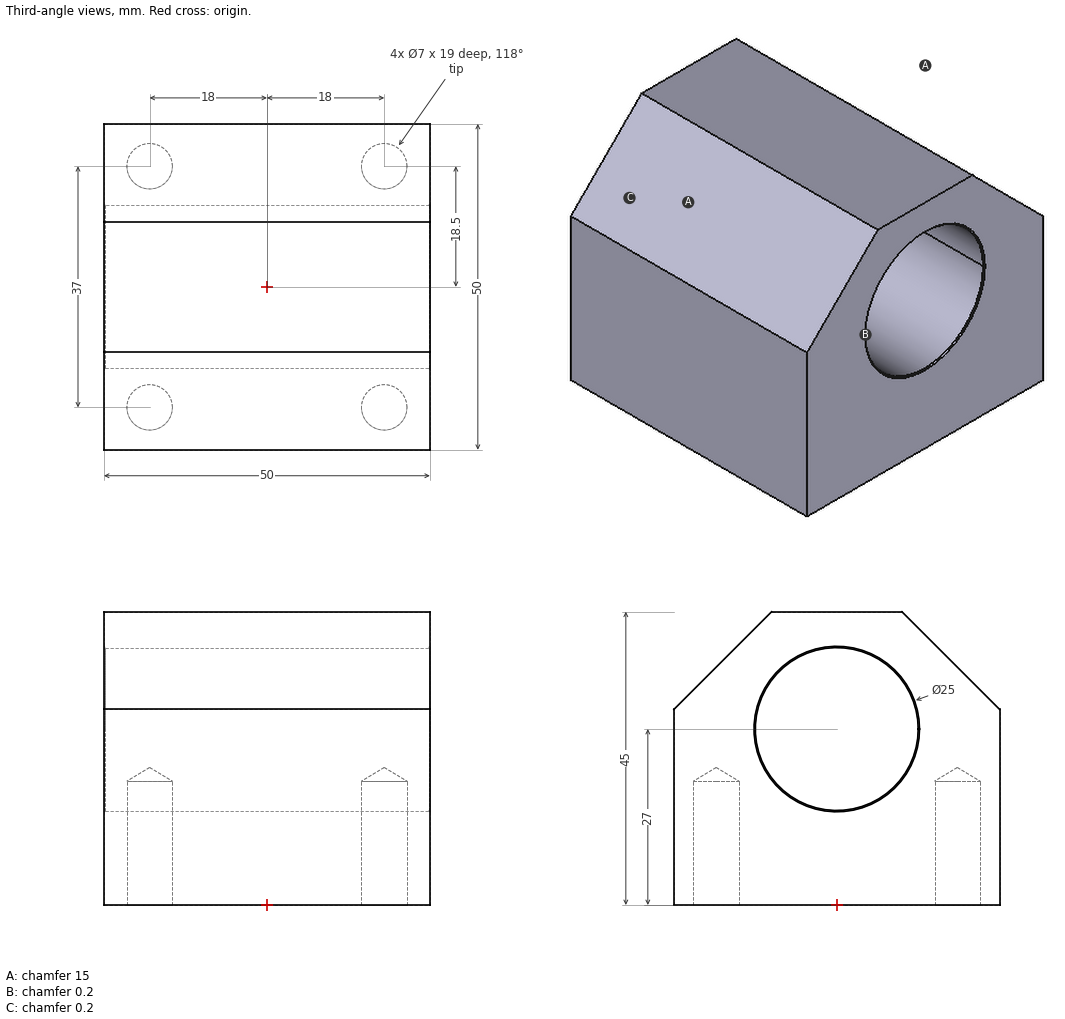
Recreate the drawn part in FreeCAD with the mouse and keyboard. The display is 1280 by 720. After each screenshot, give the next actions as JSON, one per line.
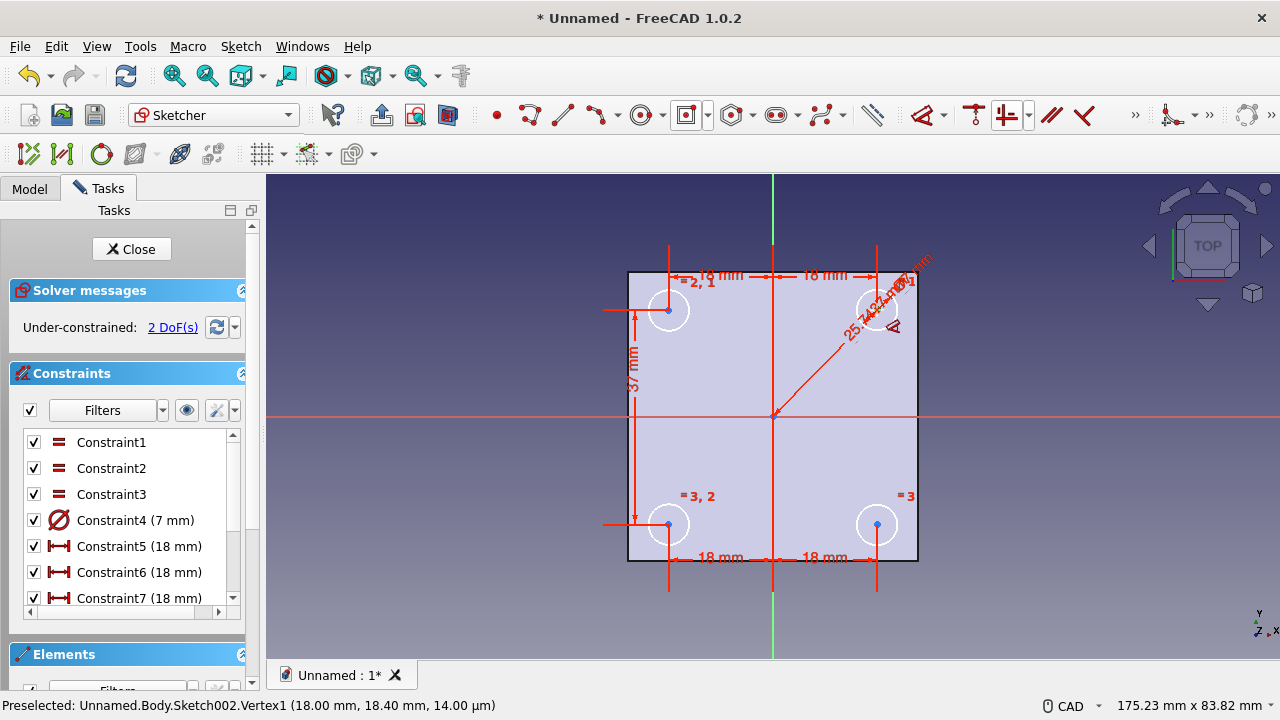
{"action": "left_click", "coordinate": [669, 525]}
{"action": "left_click", "coordinate": [911, 368]}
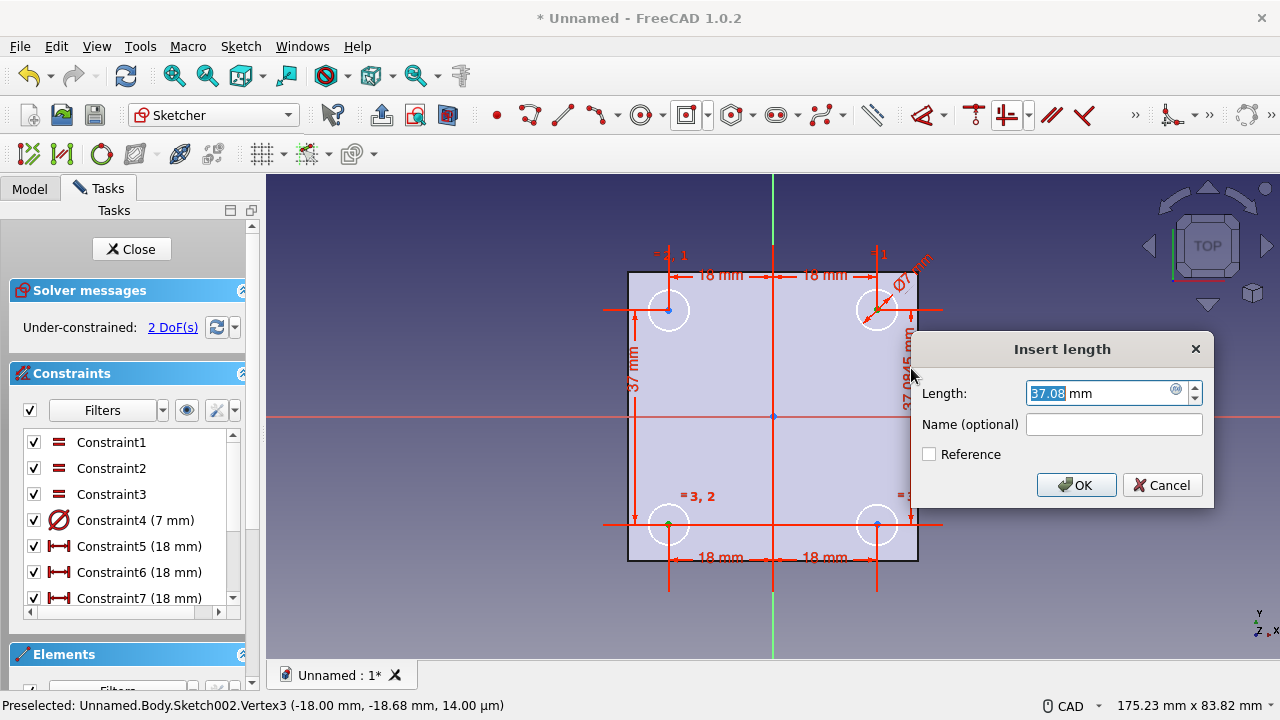
{"action": "type", "text": "37"}
{"action": "key", "text": "Return"}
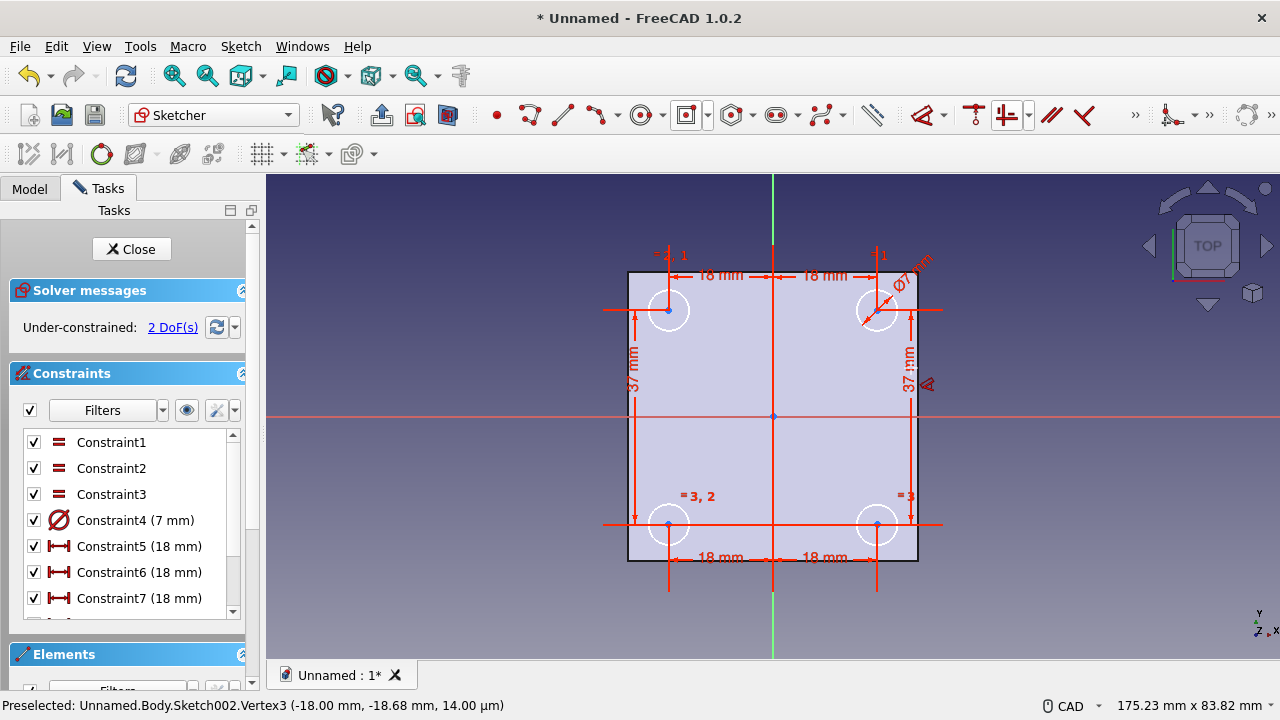
{"action": "left_click", "coordinate": [877, 310]}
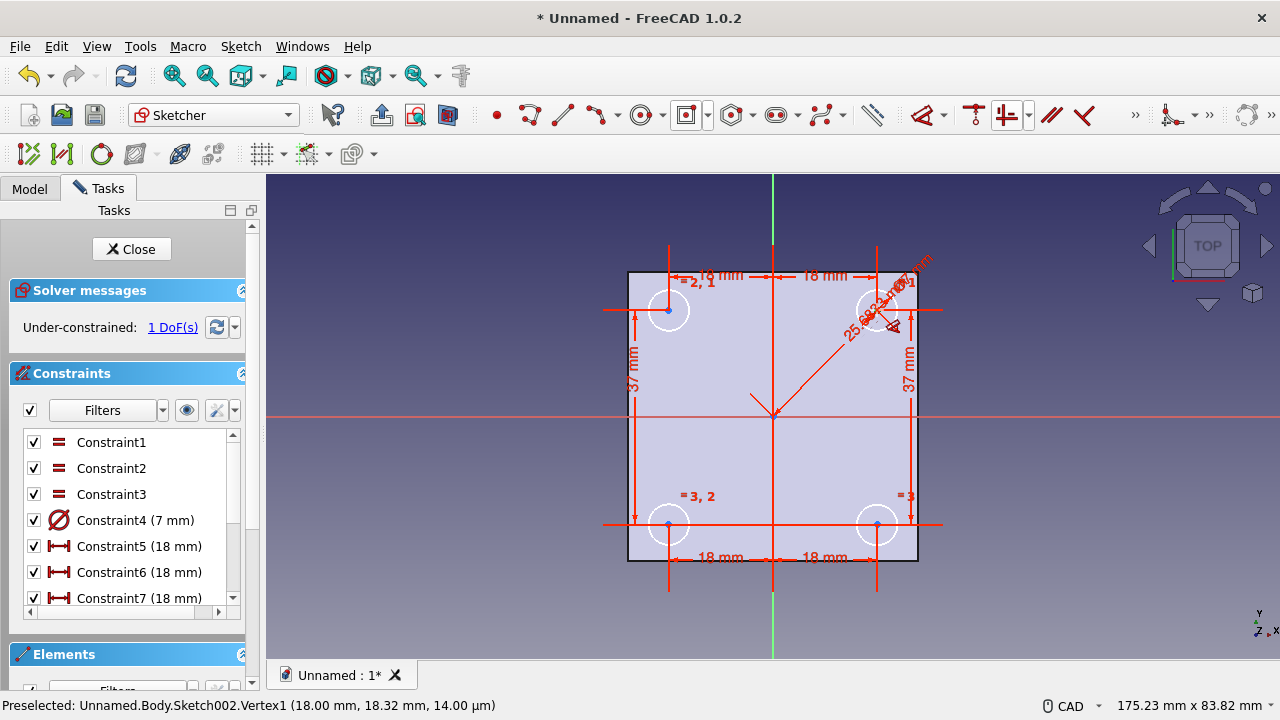
{"action": "left_click", "coordinate": [877, 525]}
{"action": "left_click", "coordinate": [911, 467]}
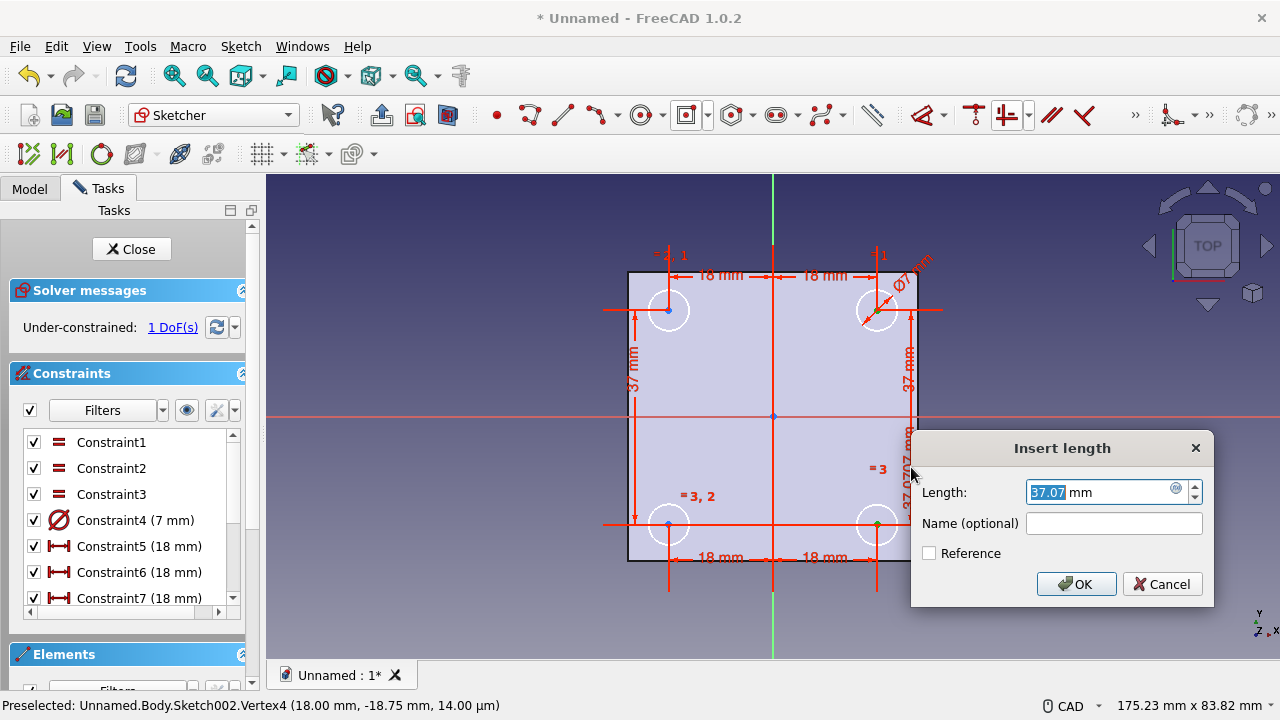
{"action": "type", "text": "37"}
{"action": "key", "text": "Return"}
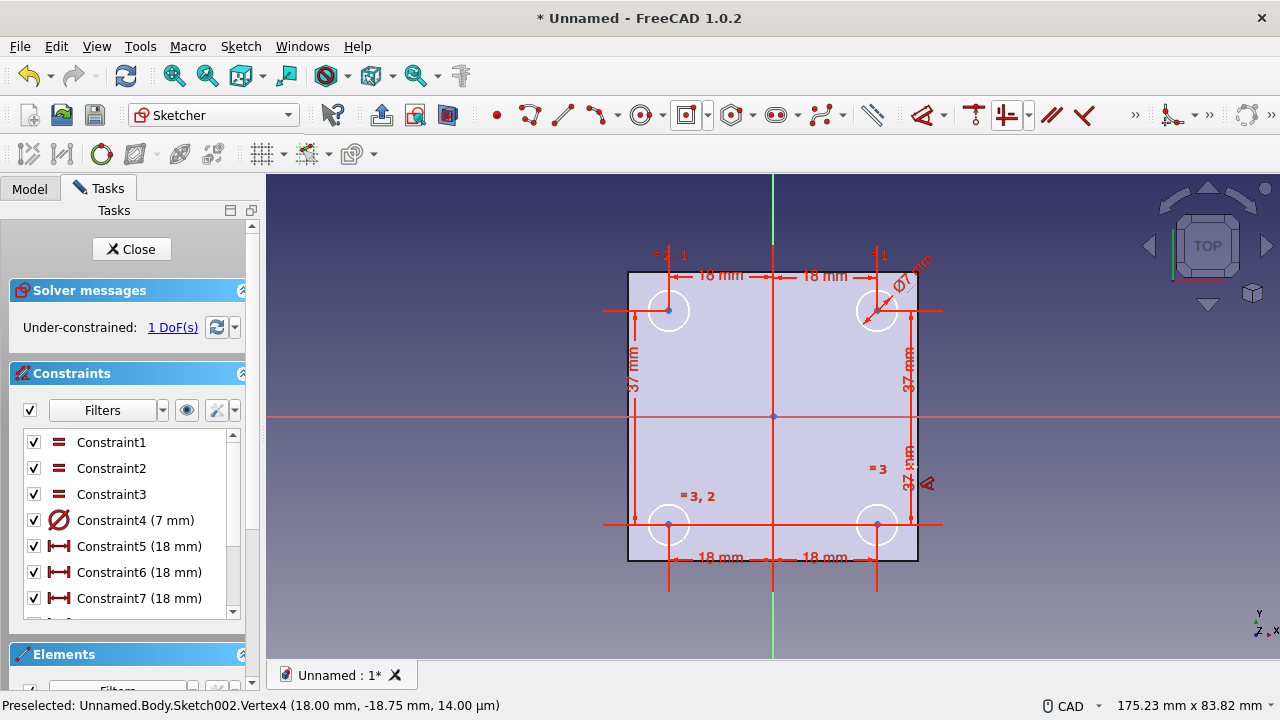
{"action": "left_click", "coordinate": [877, 311]}
{"action": "left_click", "coordinate": [911, 339]}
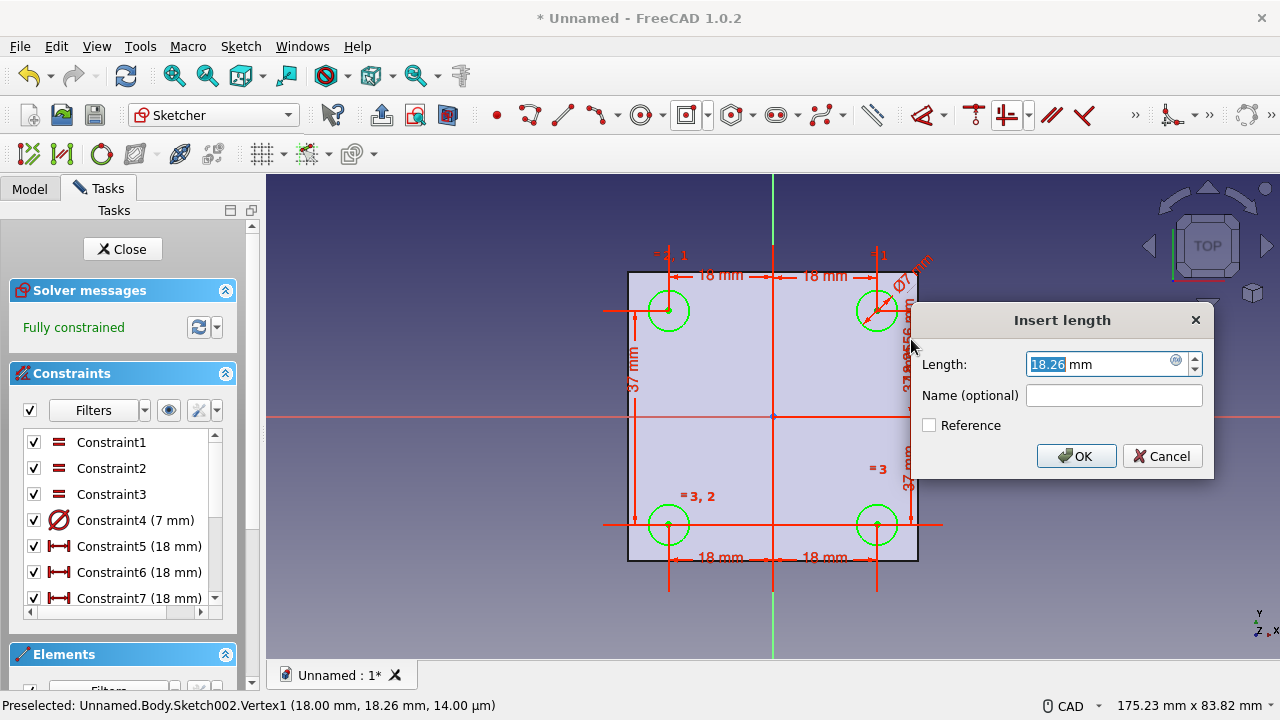
{"action": "type", "text": "18.5"}
{"action": "key", "text": "Return"}
{"action": "key", "text": "Escape"}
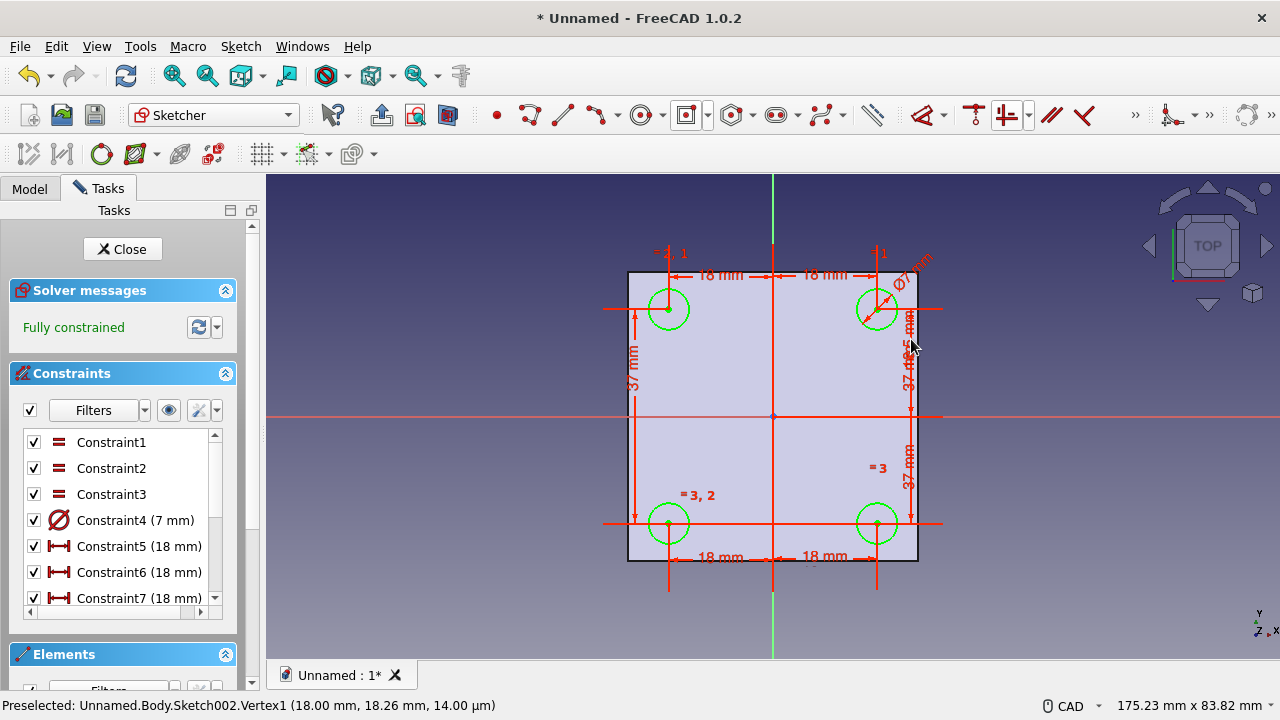
{"action": "left_click", "coordinate": [123, 249]}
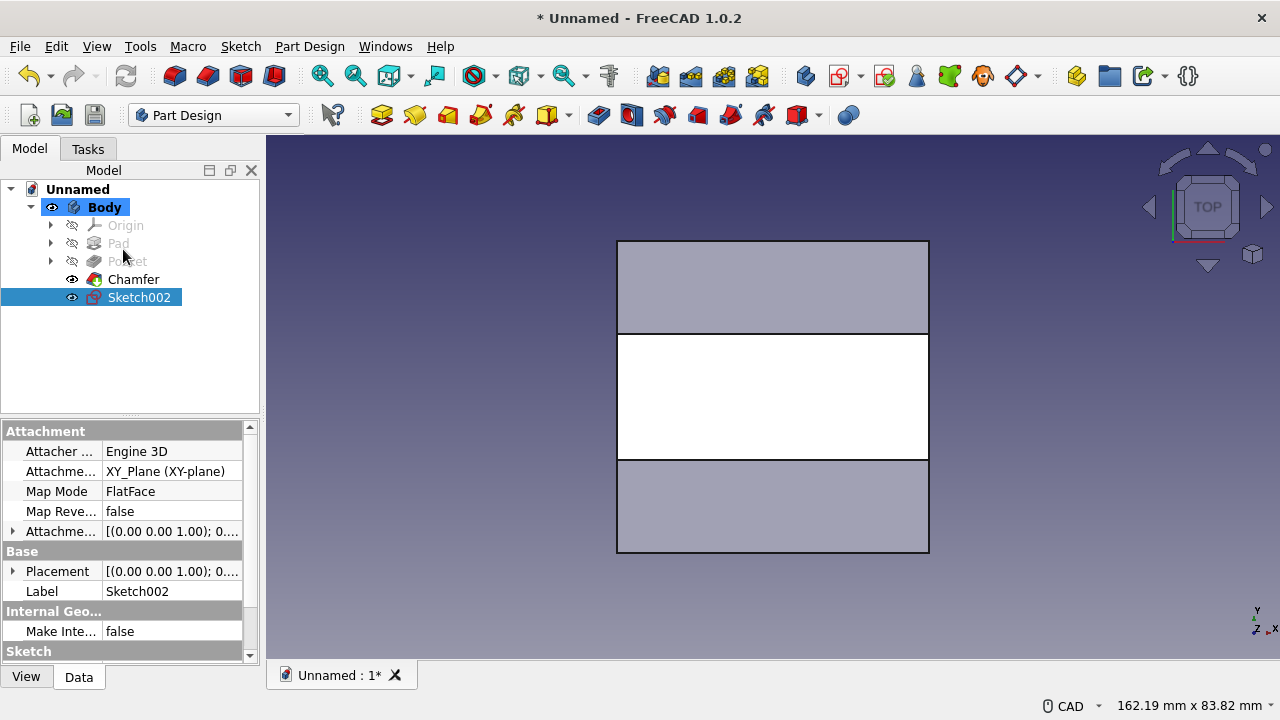
{"action": "left_click", "coordinate": [632, 116]}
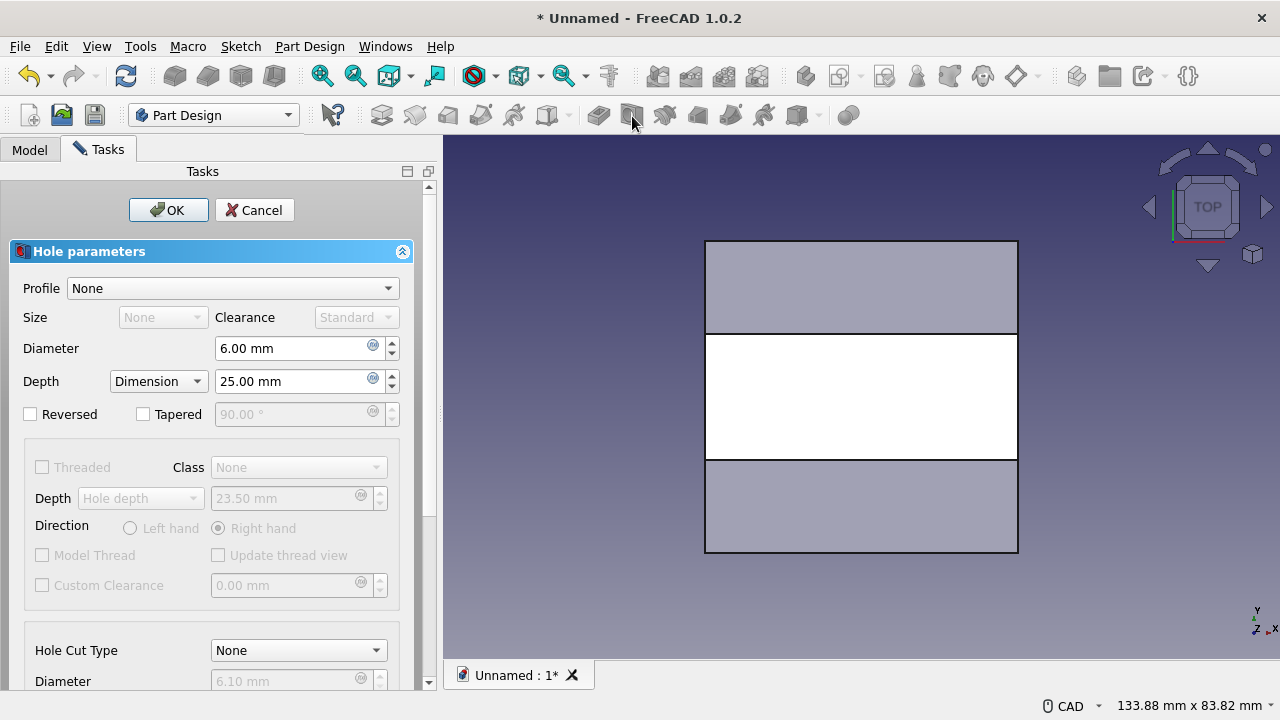
{"action": "triple_click", "coordinate": [300, 348]}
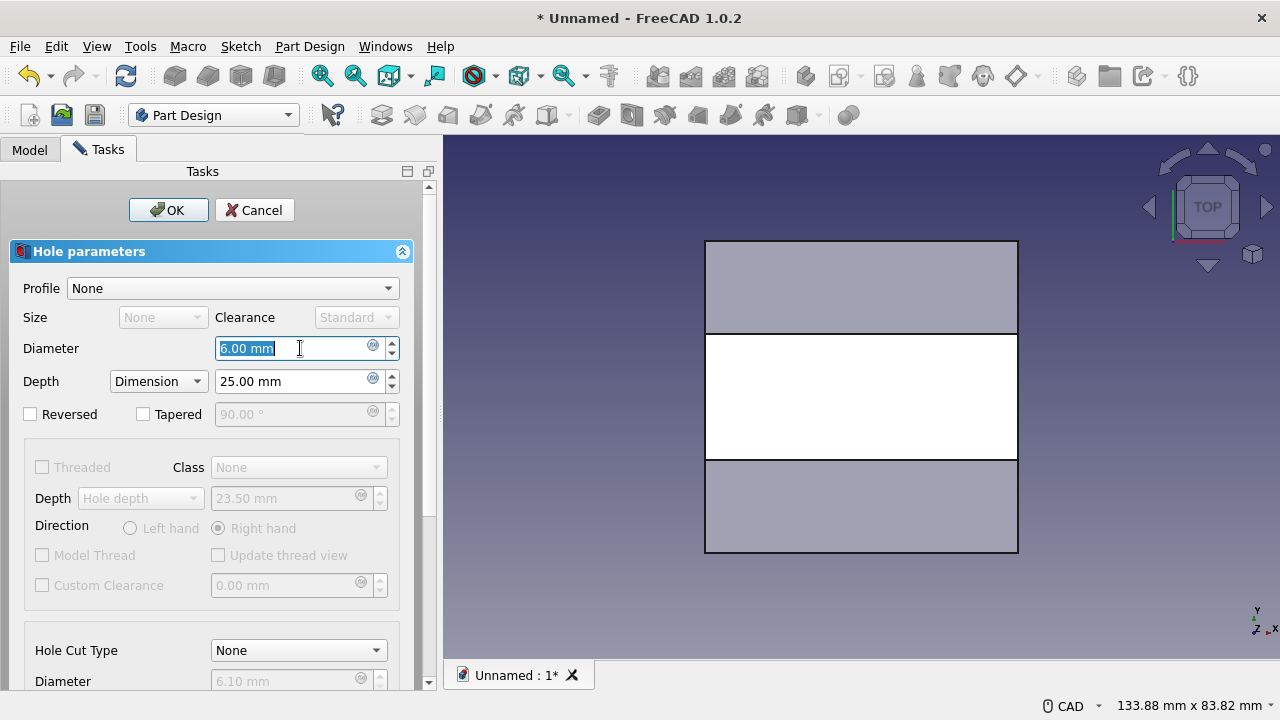
{"action": "type", "text": "7"}
{"action": "key", "text": "Tab"}